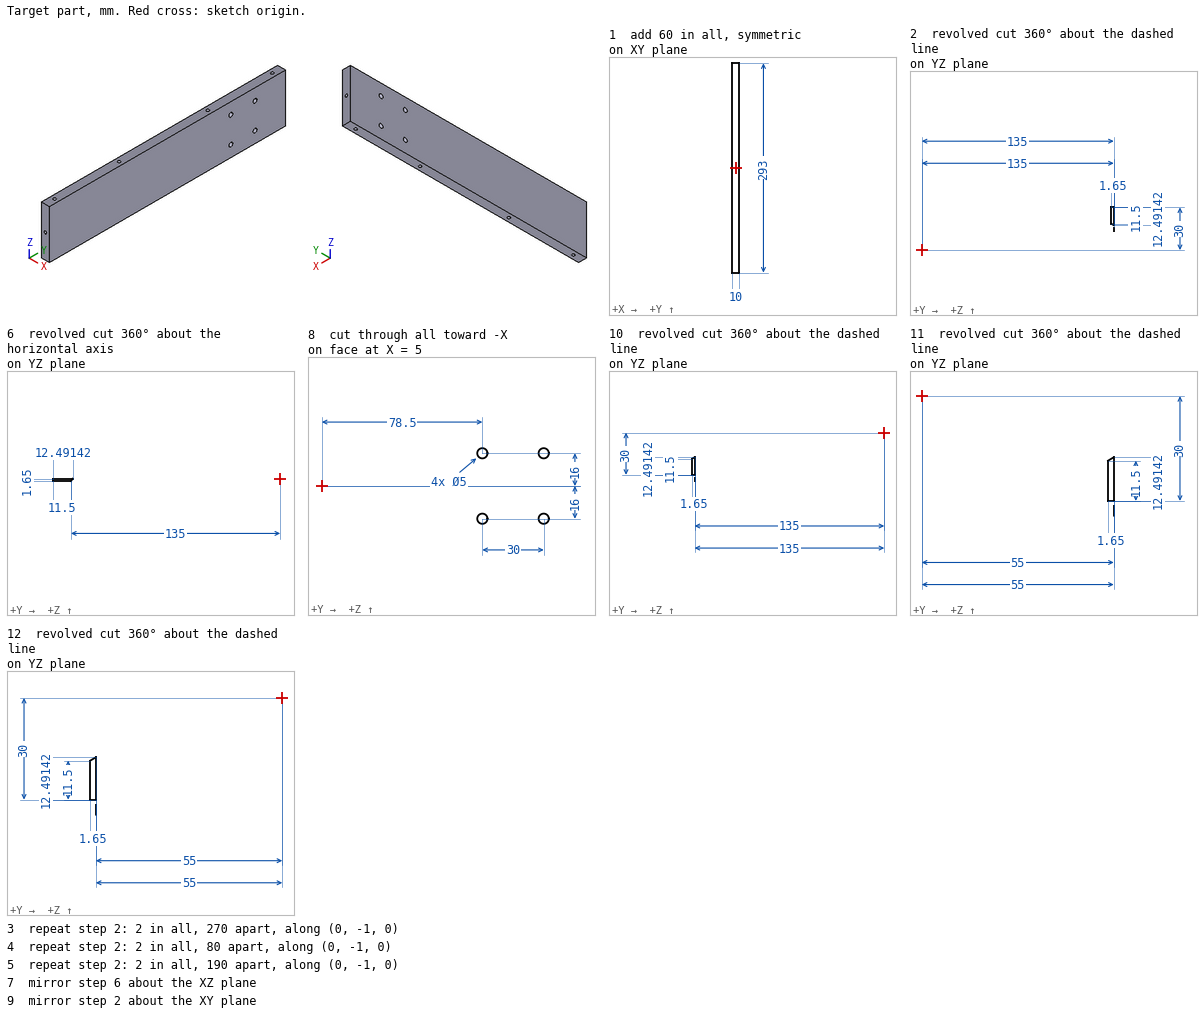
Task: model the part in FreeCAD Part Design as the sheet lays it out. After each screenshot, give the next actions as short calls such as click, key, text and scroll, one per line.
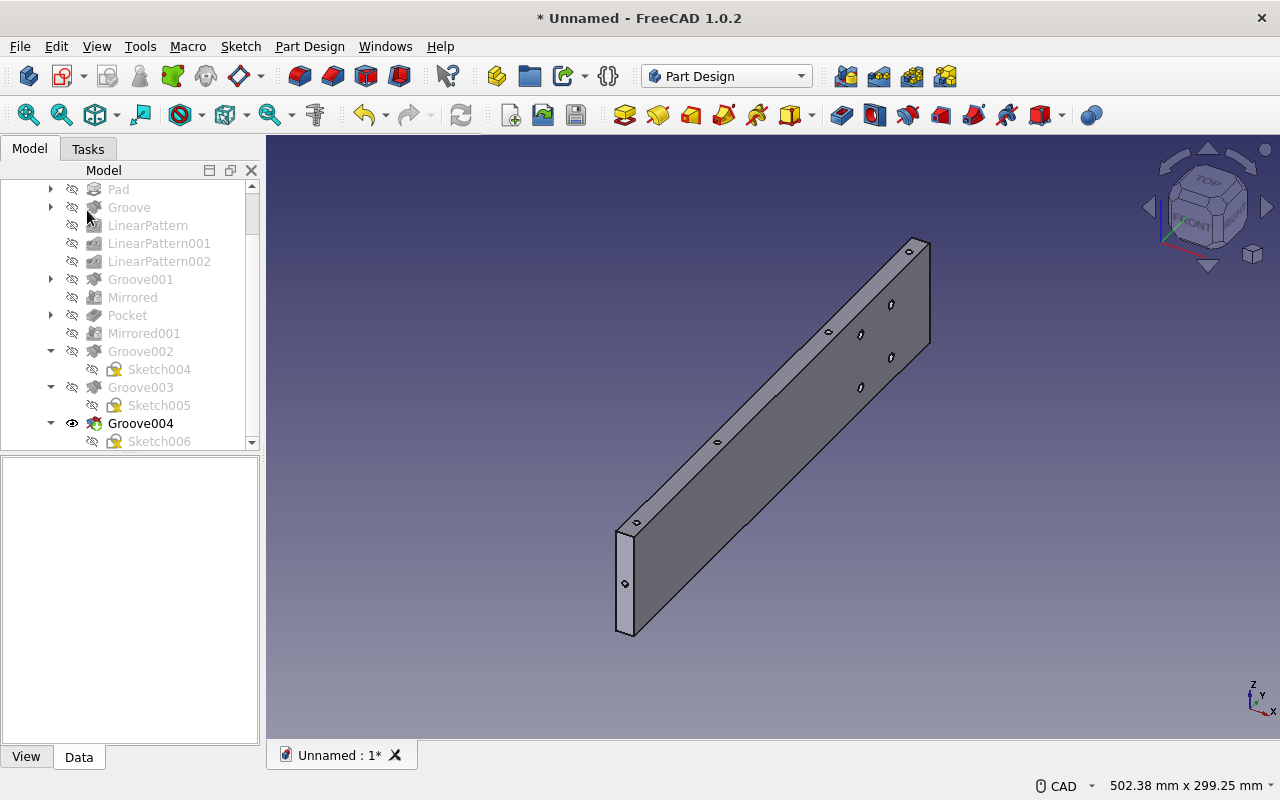
key(0)